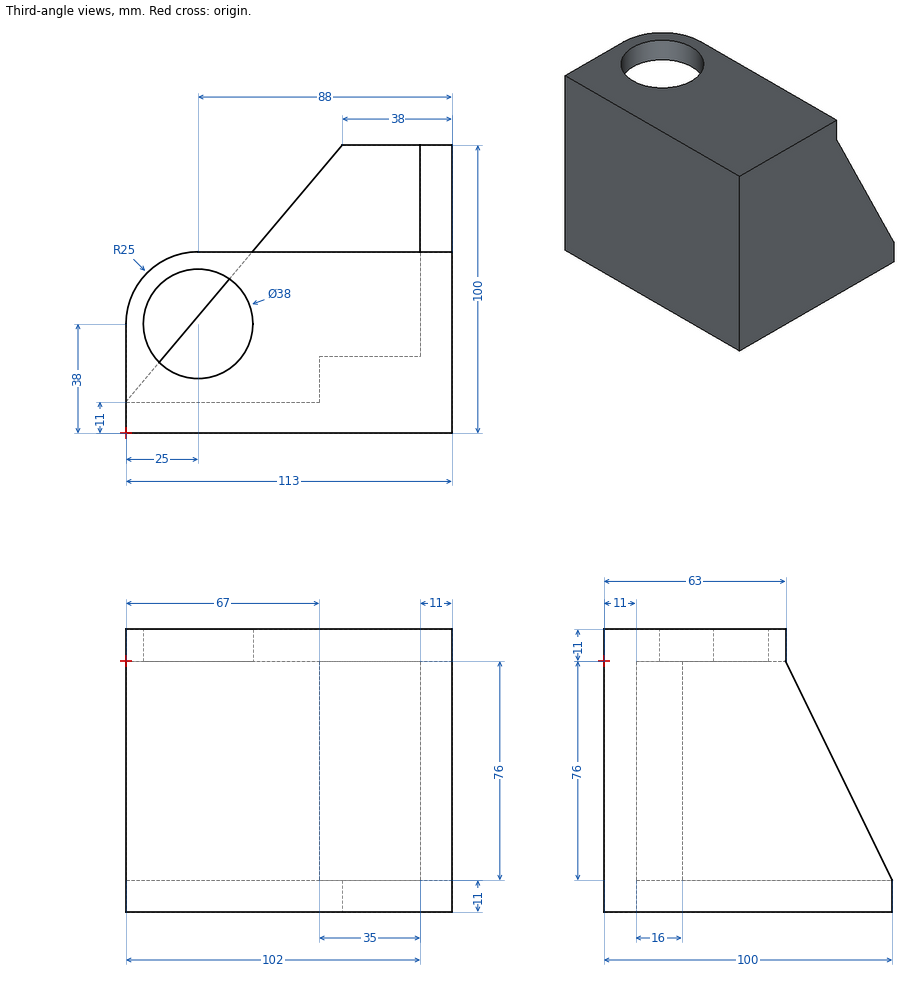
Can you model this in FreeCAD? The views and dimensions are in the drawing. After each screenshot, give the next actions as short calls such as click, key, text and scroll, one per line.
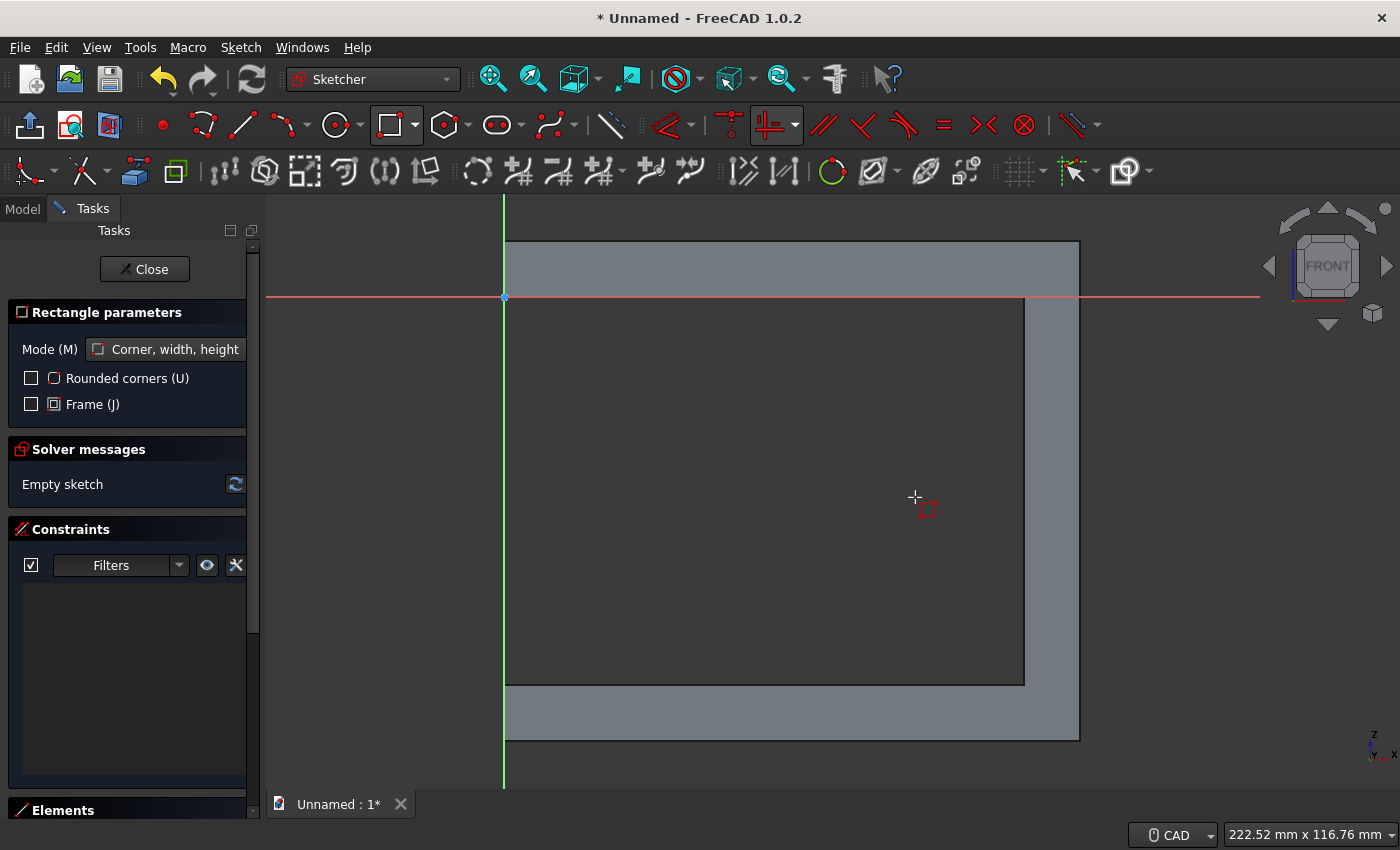
click(504, 297)
move(1024, 685)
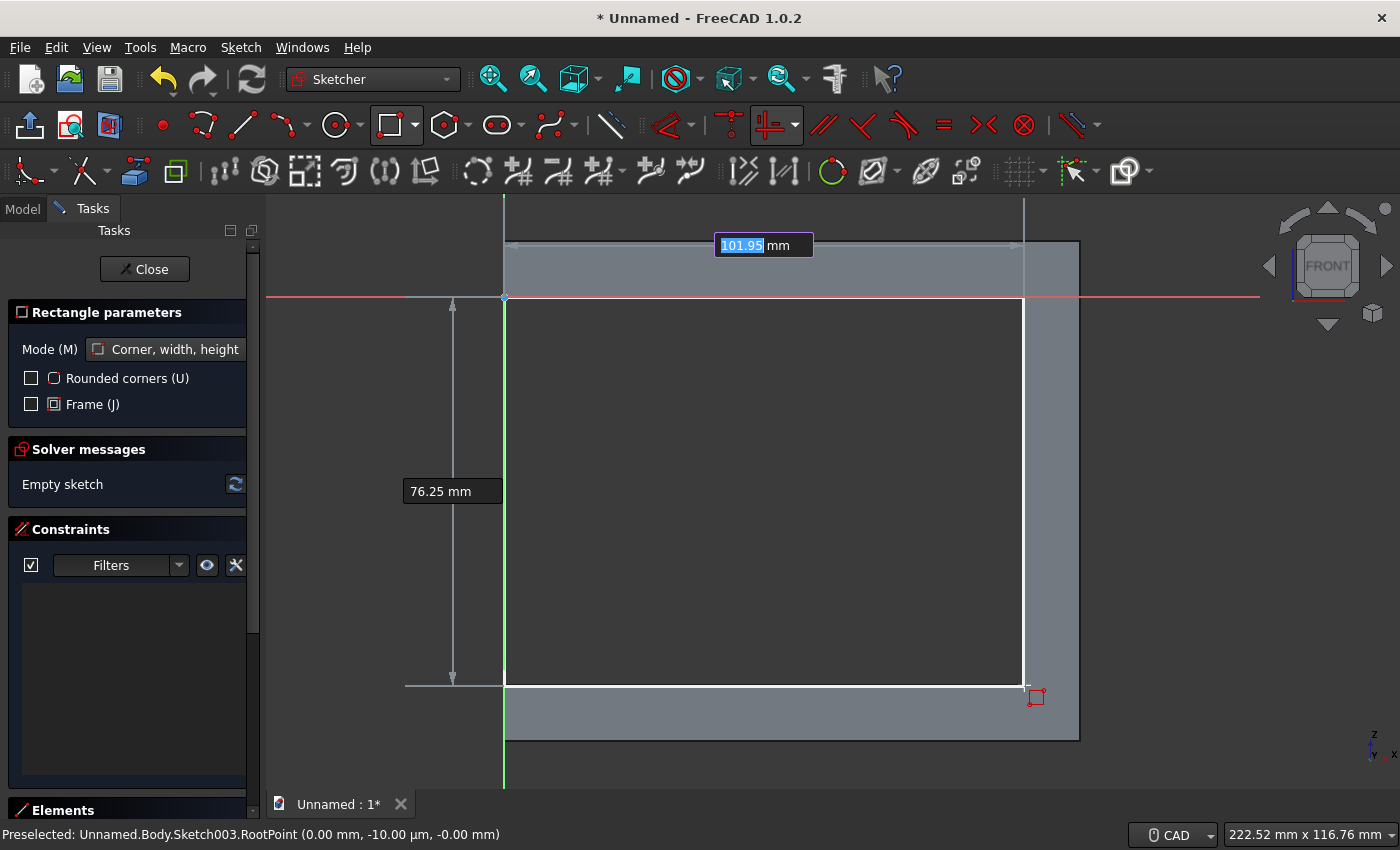
text(102)
key(Tab)
text(76)
key(Return)
key(Escape)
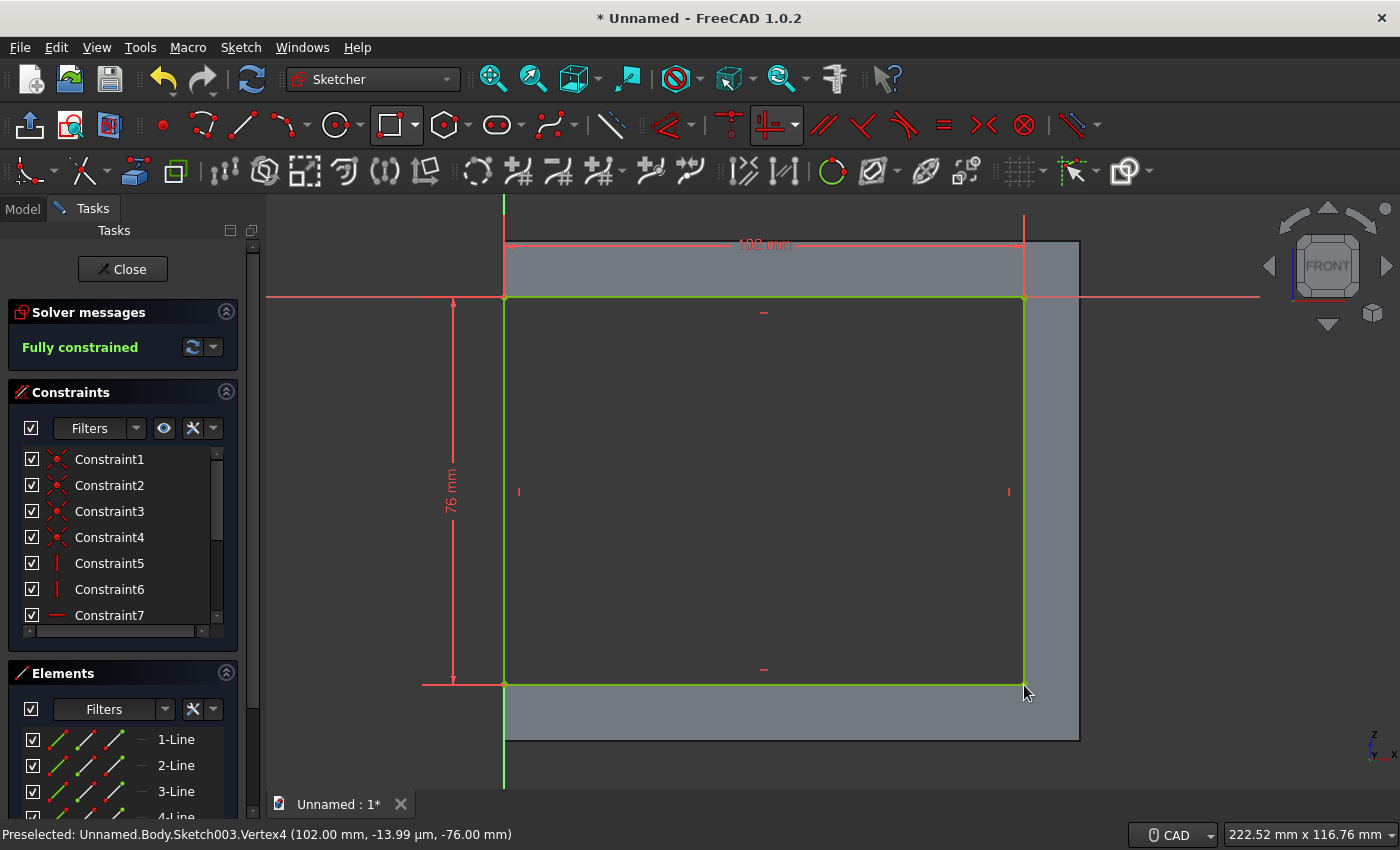
click(123, 269)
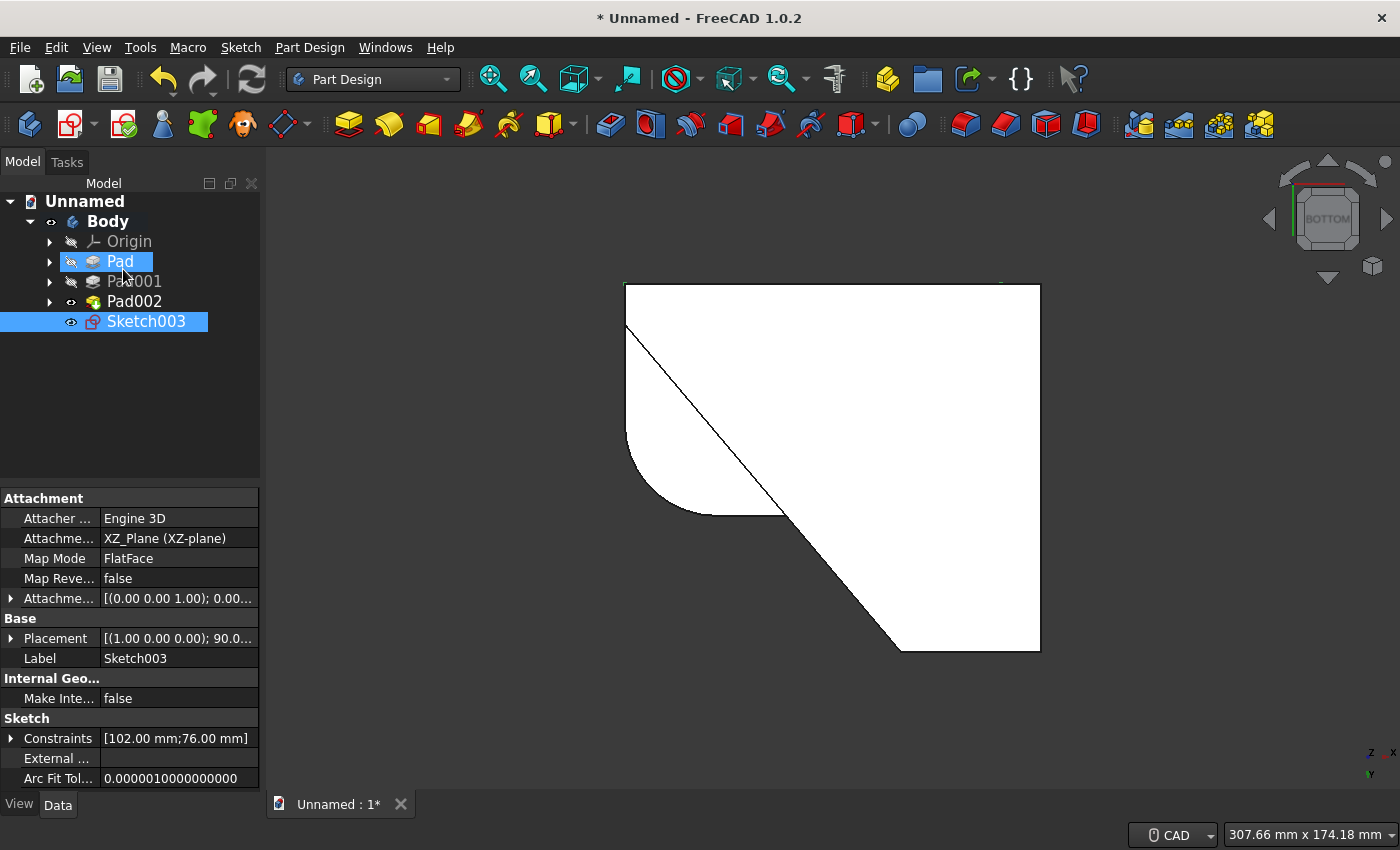
click(350, 124)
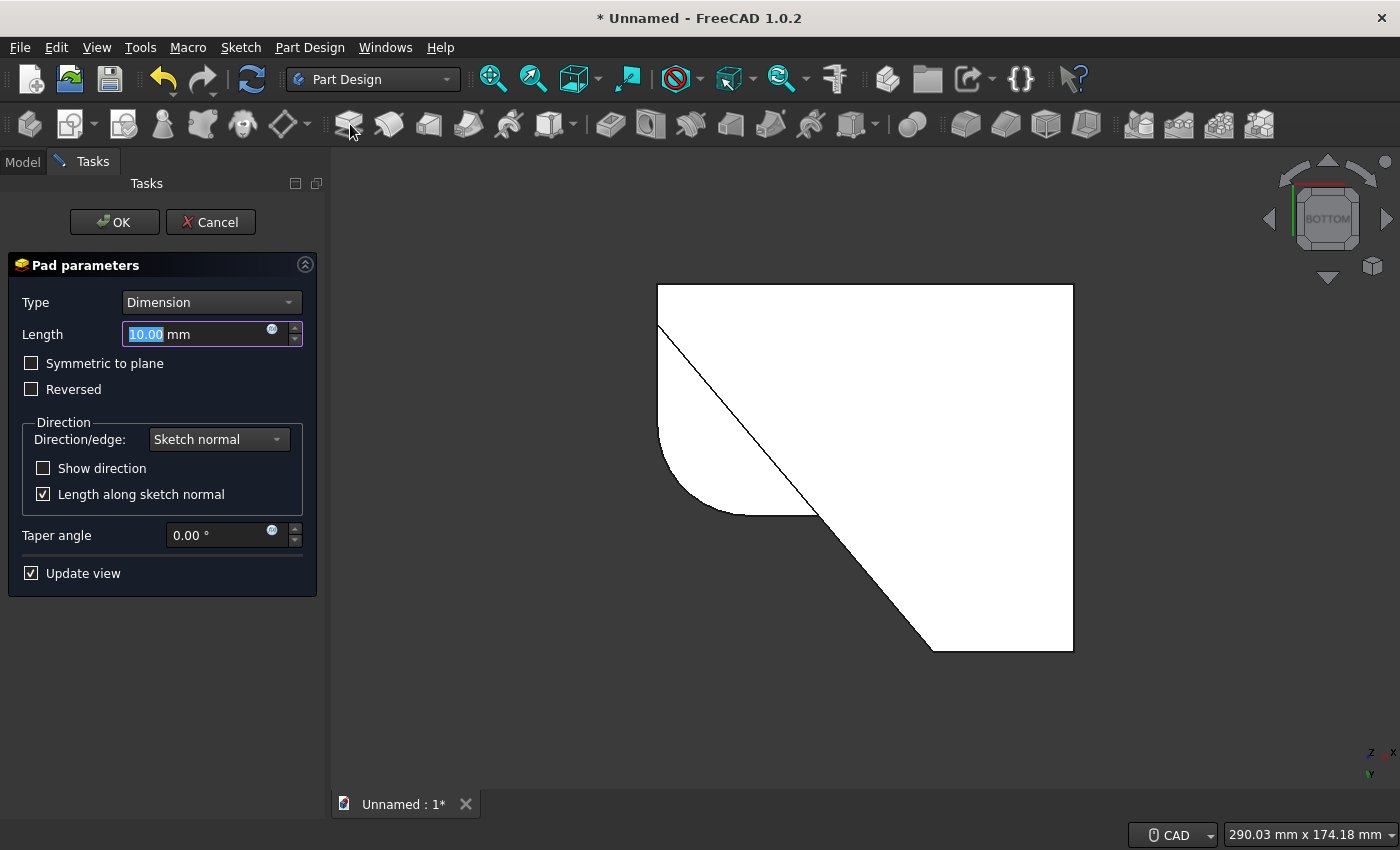
text(11)
key(Tab)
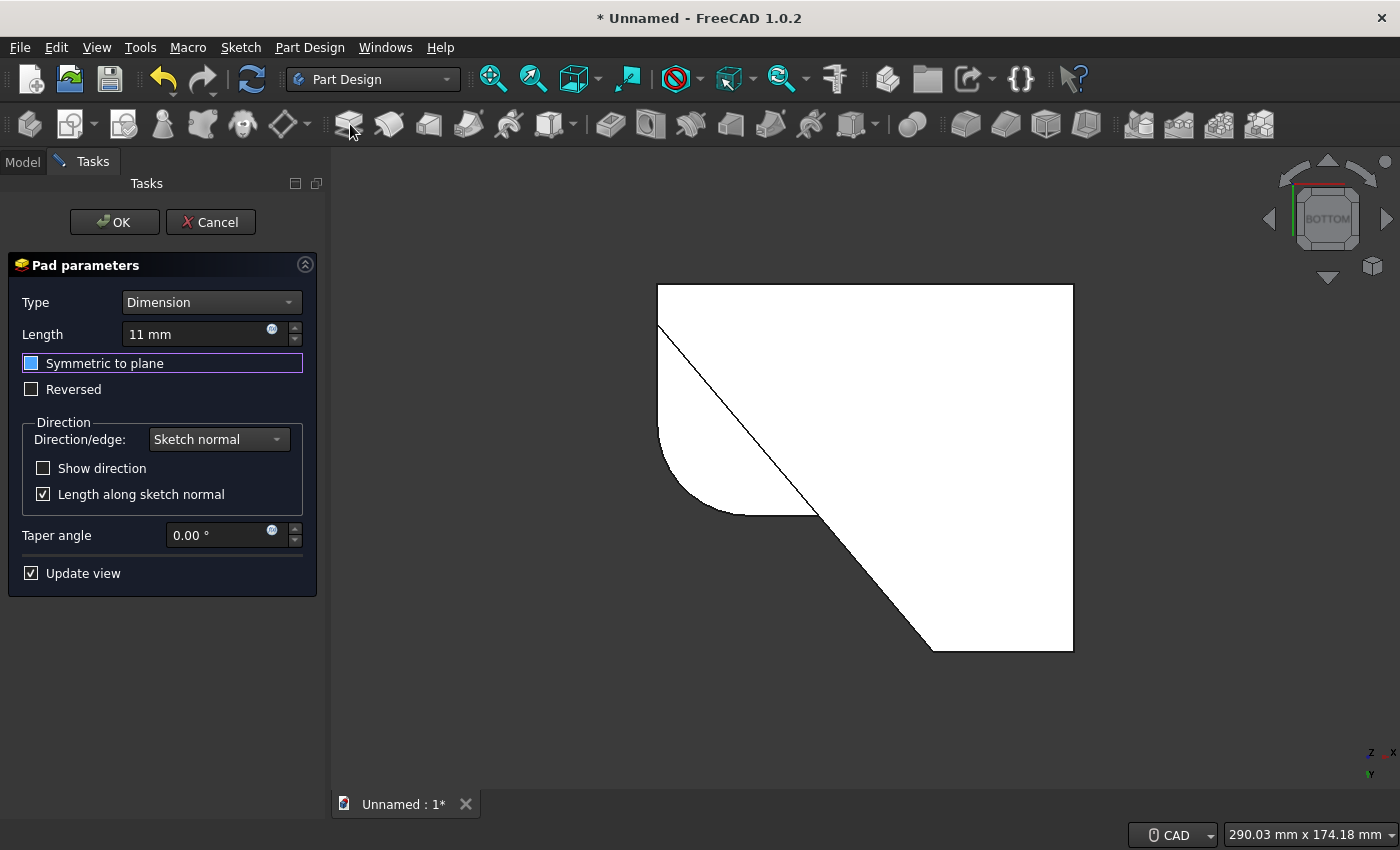
click(30, 389)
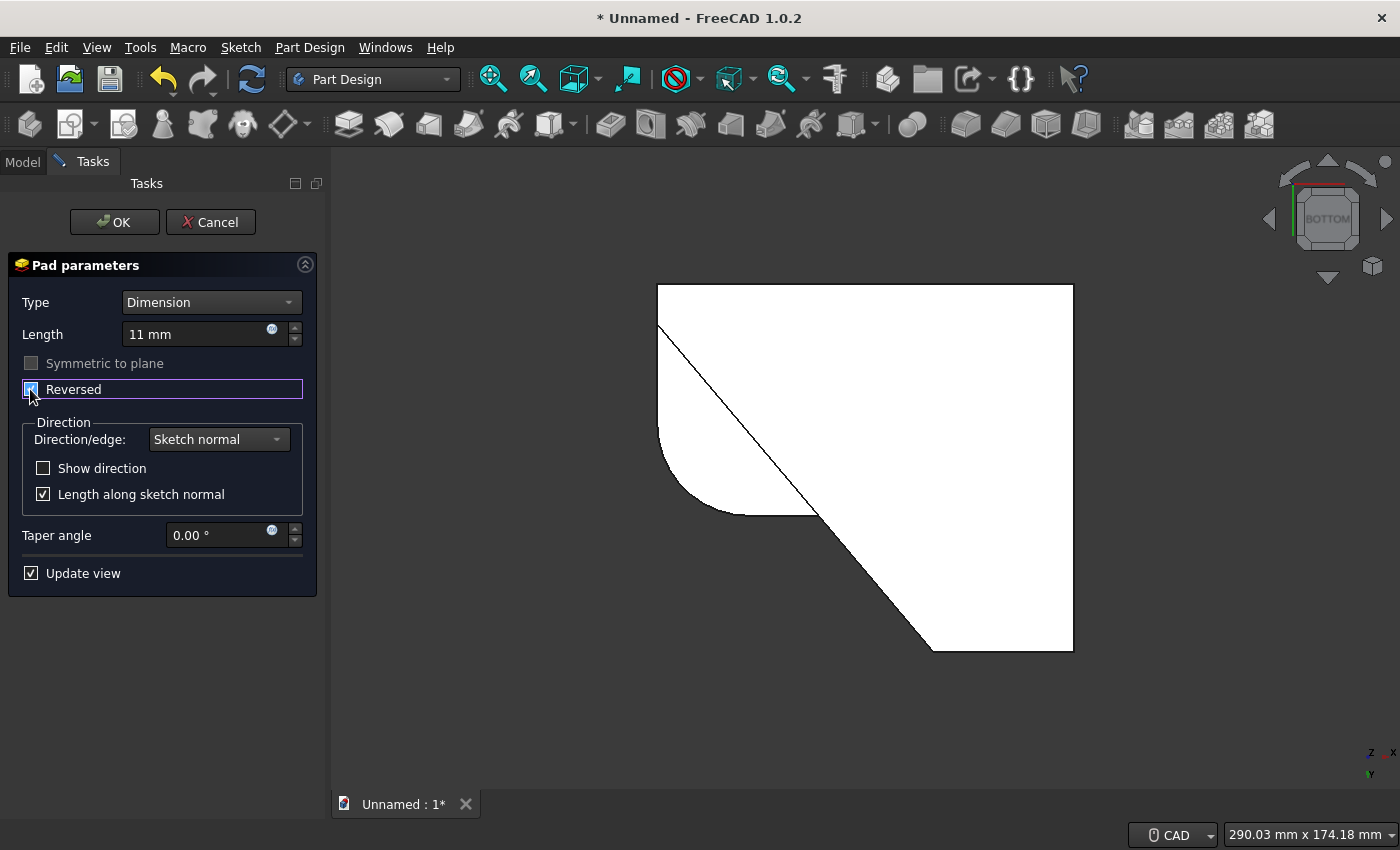
click(115, 222)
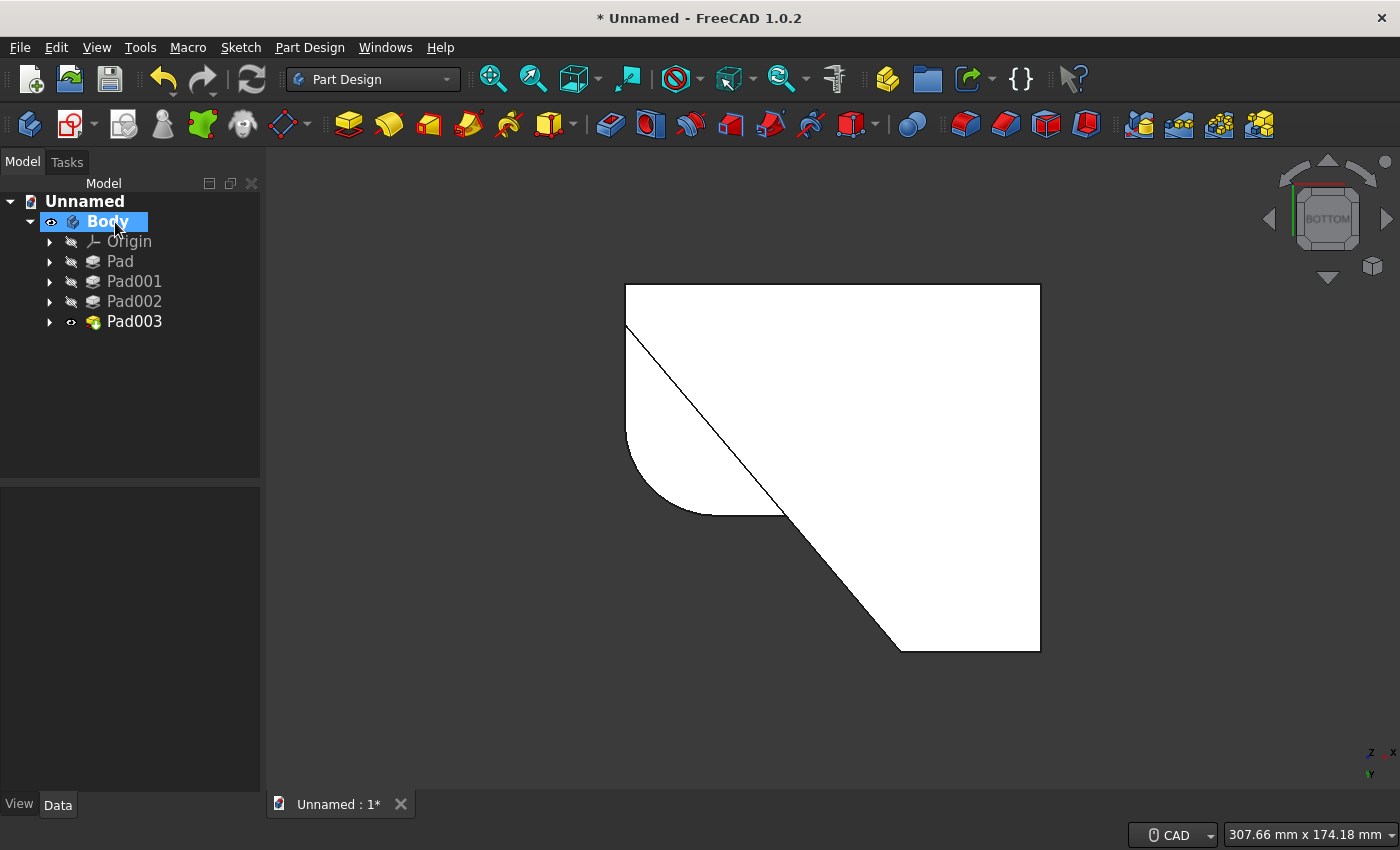
key(4)